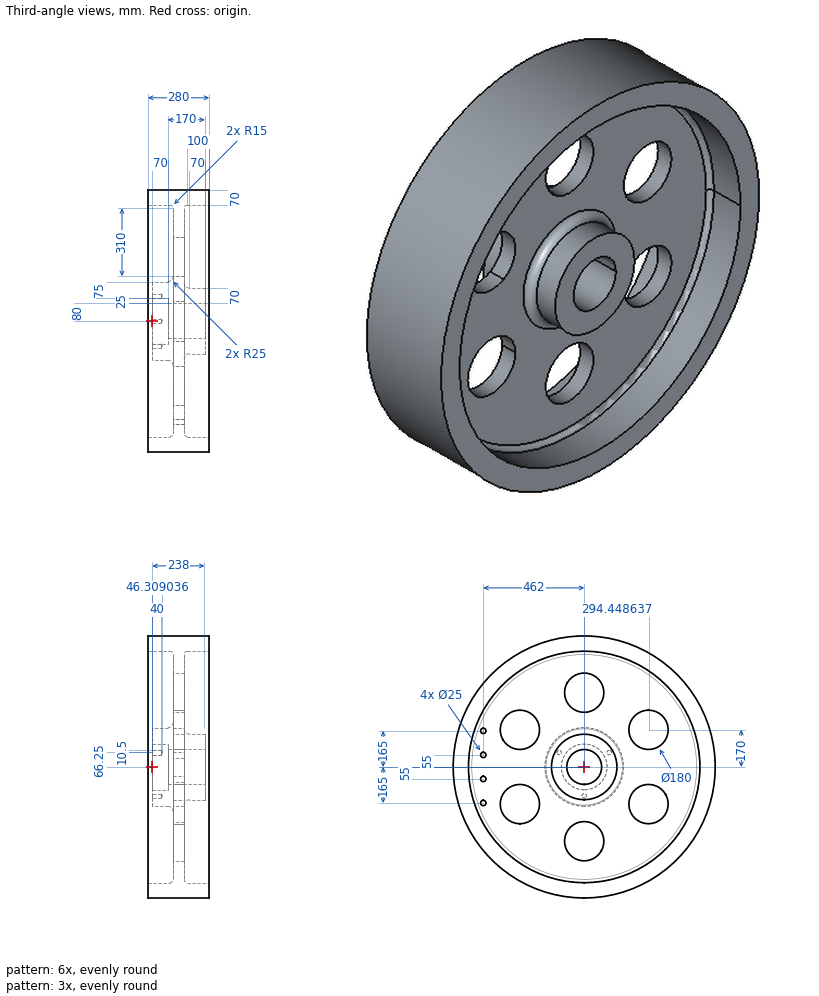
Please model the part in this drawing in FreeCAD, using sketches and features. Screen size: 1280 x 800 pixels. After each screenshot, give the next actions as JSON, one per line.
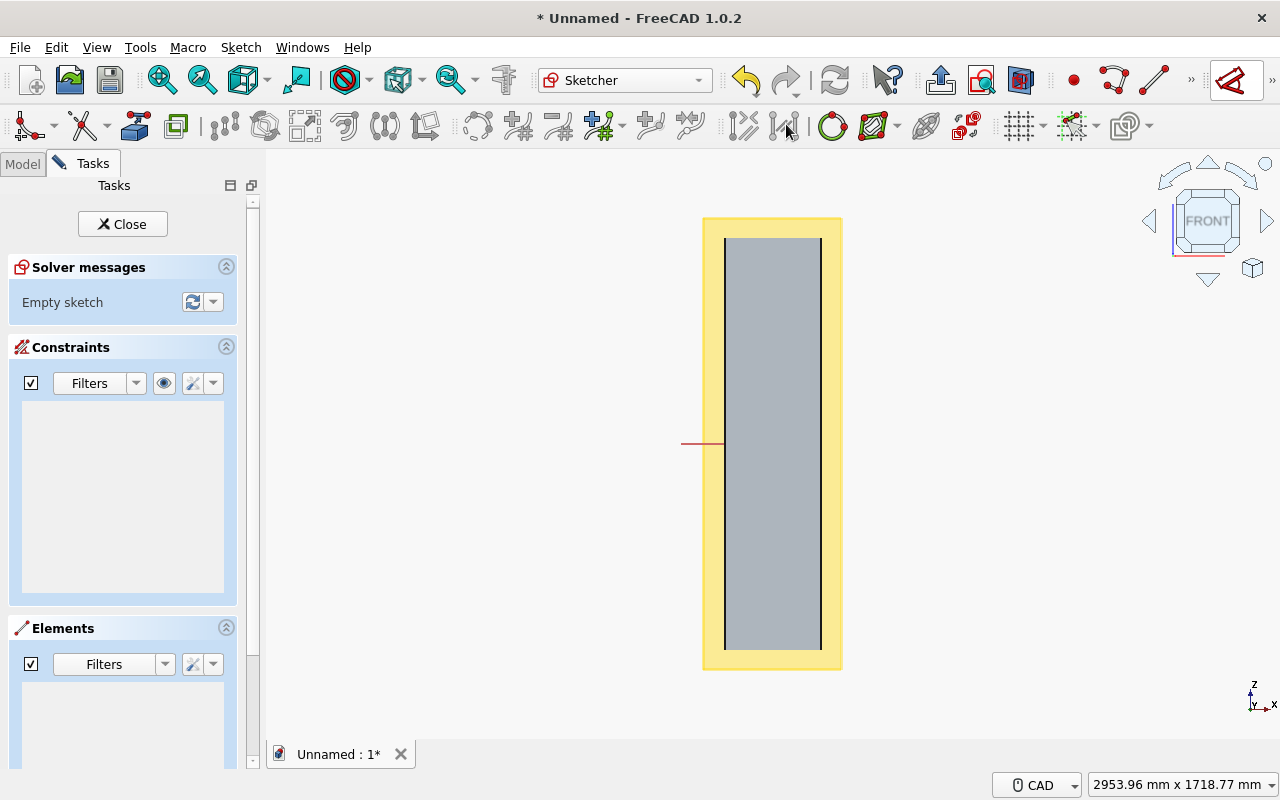
{"action": "left_click", "coordinate": [1022, 80]}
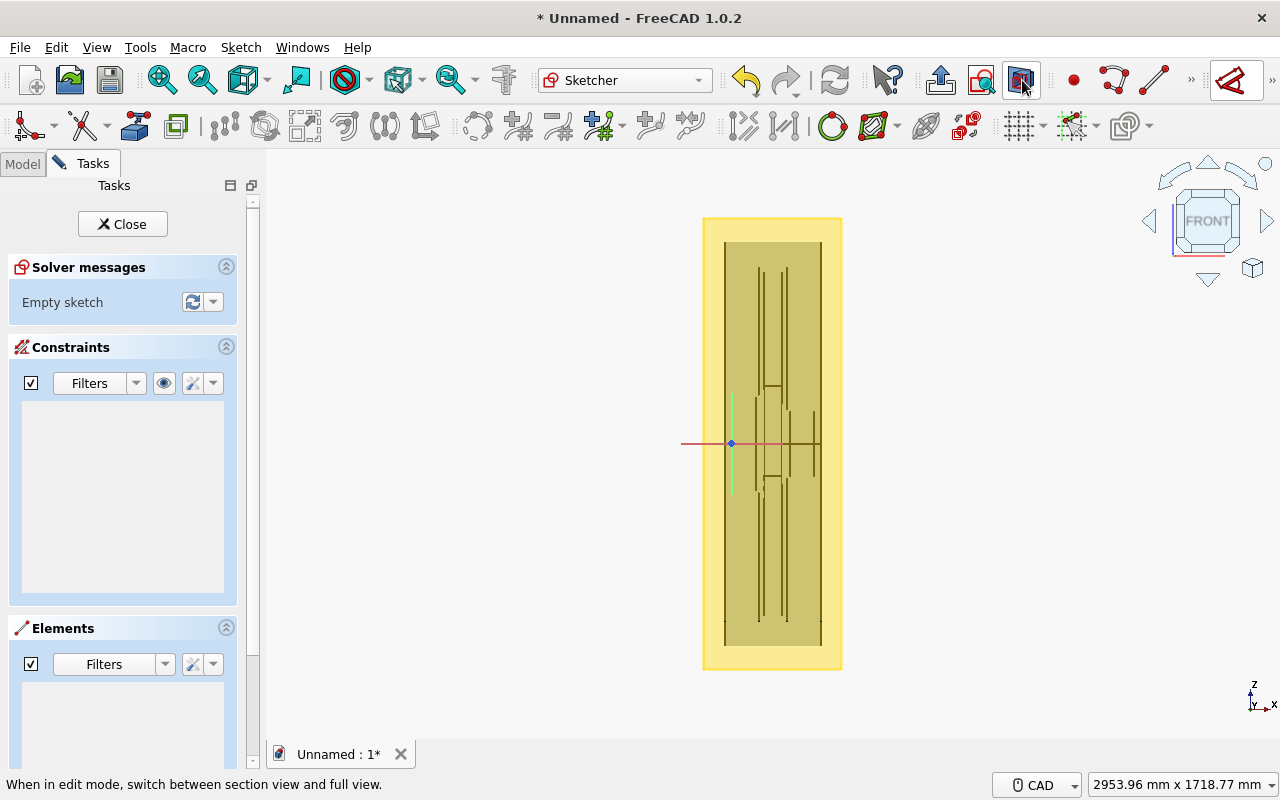
{"action": "scroll", "coordinate": [746, 430], "scroll_direction": "up", "scroll_amount": 13}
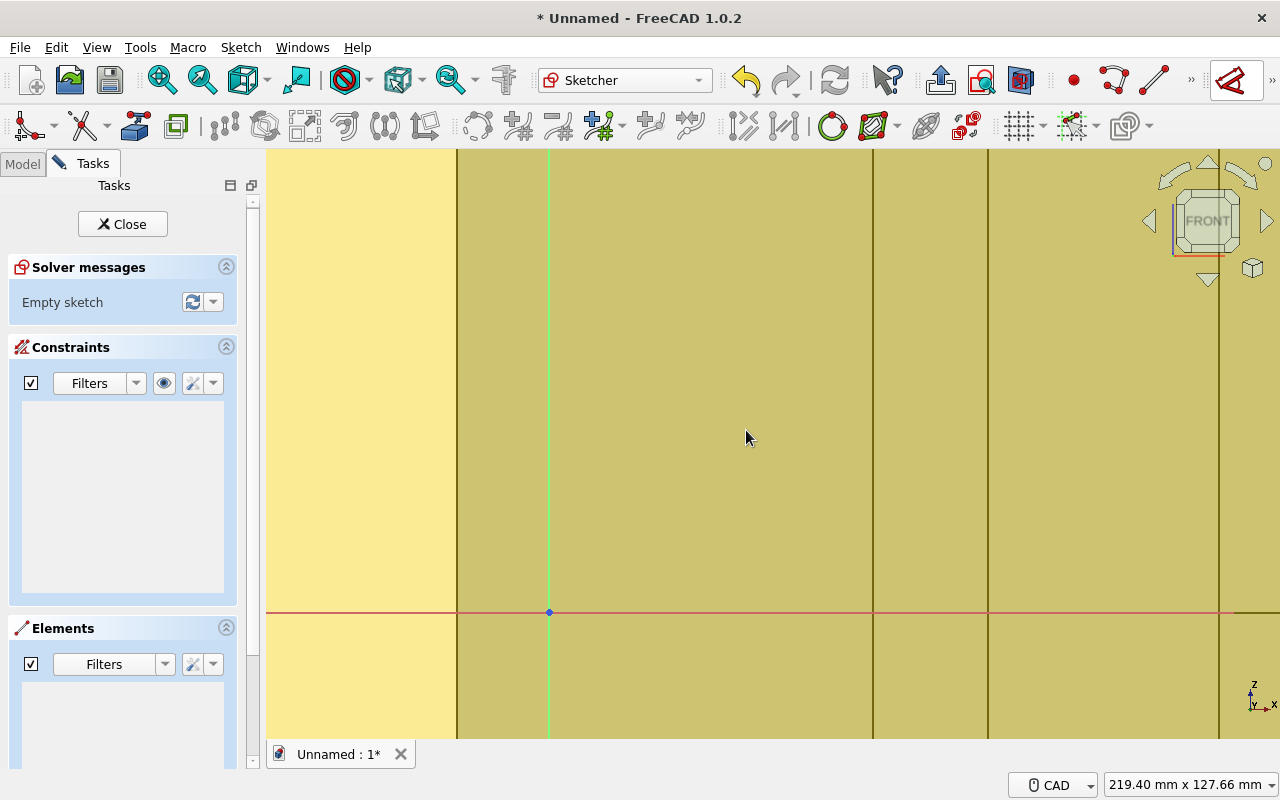
{"action": "left_click", "coordinate": [1114, 80]}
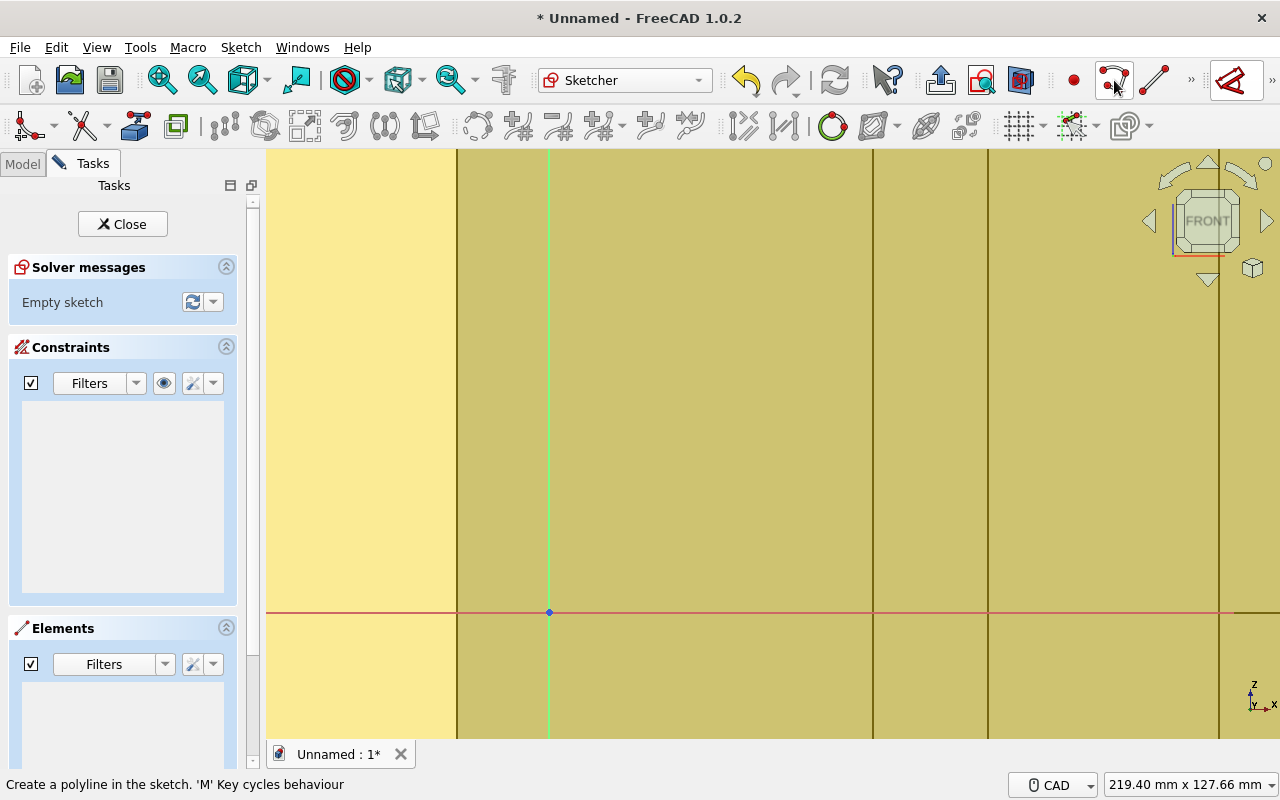
{"action": "left_click", "coordinate": [549, 306]}
{"action": "left_click", "coordinate": [558, 258]}
{"action": "left_click", "coordinate": [734, 258]}
{"action": "left_click", "coordinate": [763, 306]}
{"action": "left_click", "coordinate": [549, 307]}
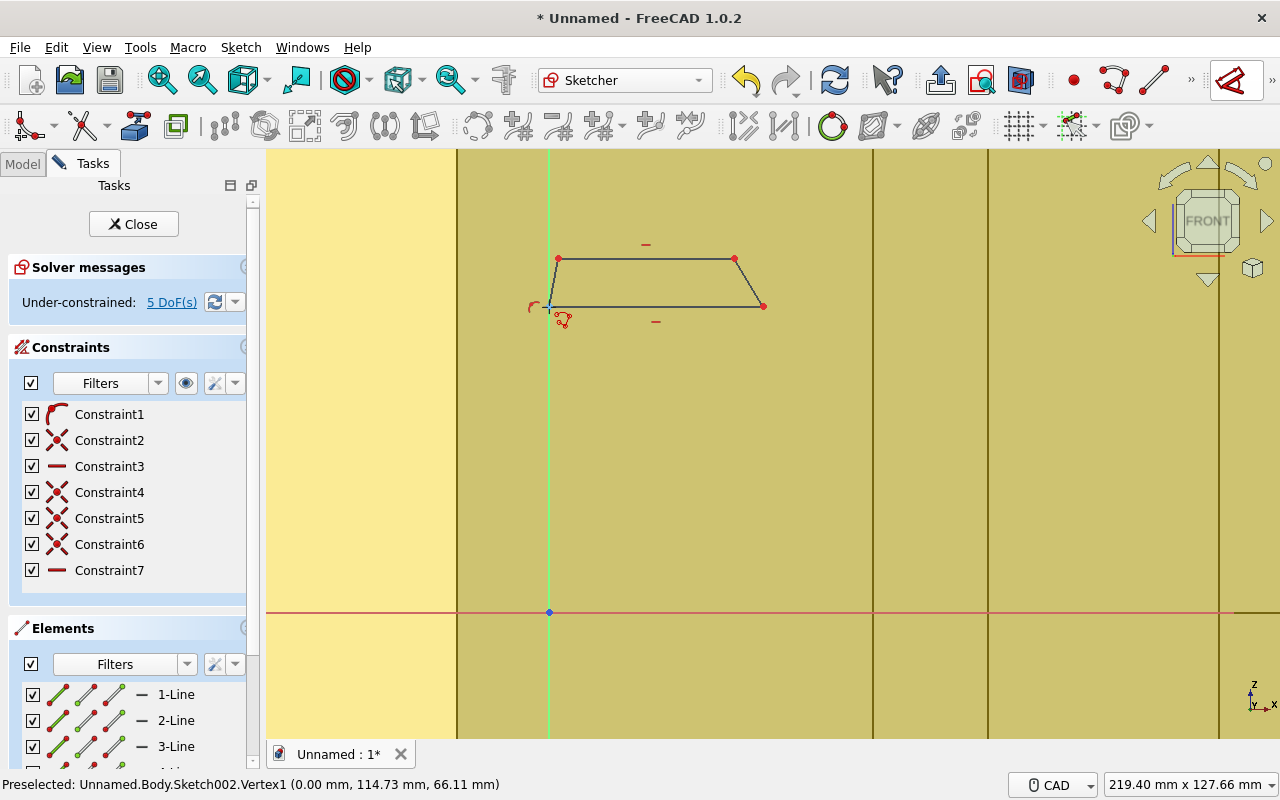
{"action": "left_click", "coordinate": [1154, 80]}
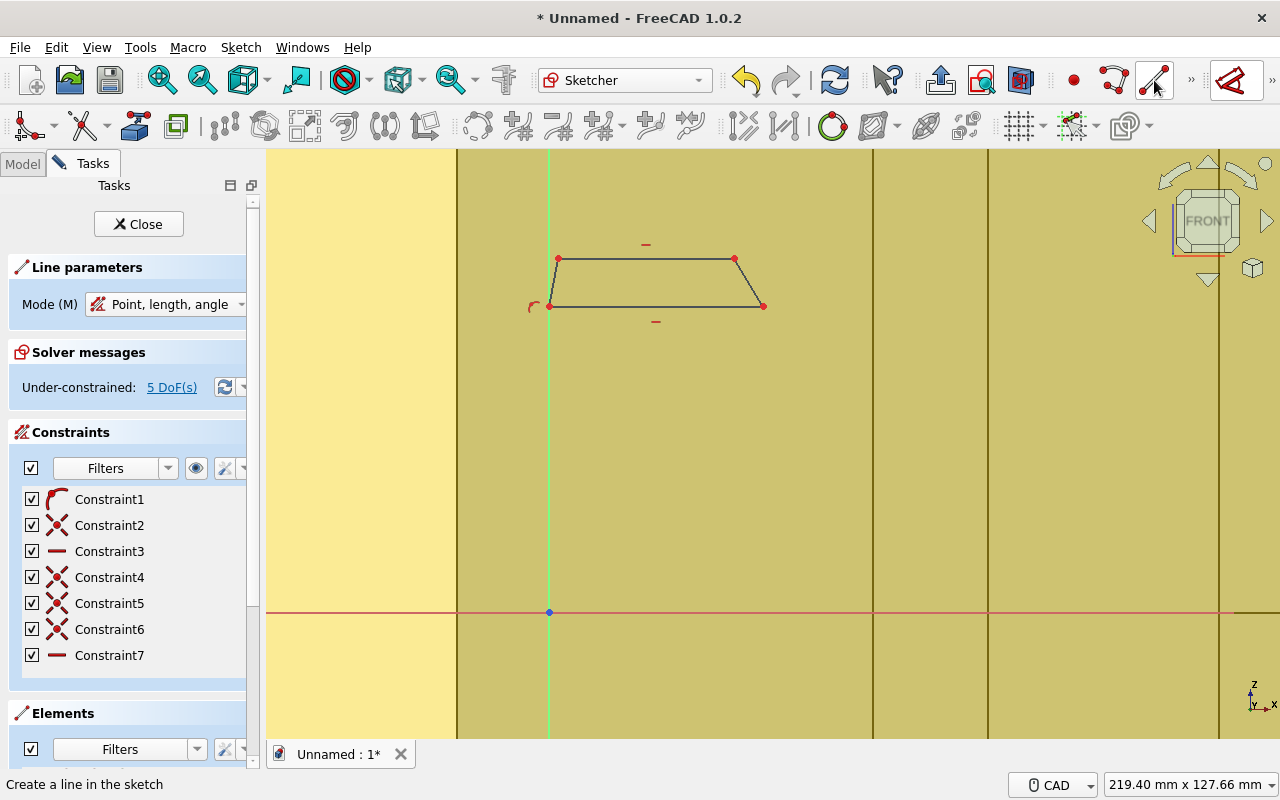
{"action": "left_click", "coordinate": [784, 306]}
{"action": "left_click", "coordinate": [849, 306]}
{"action": "key", "text": "Escape"}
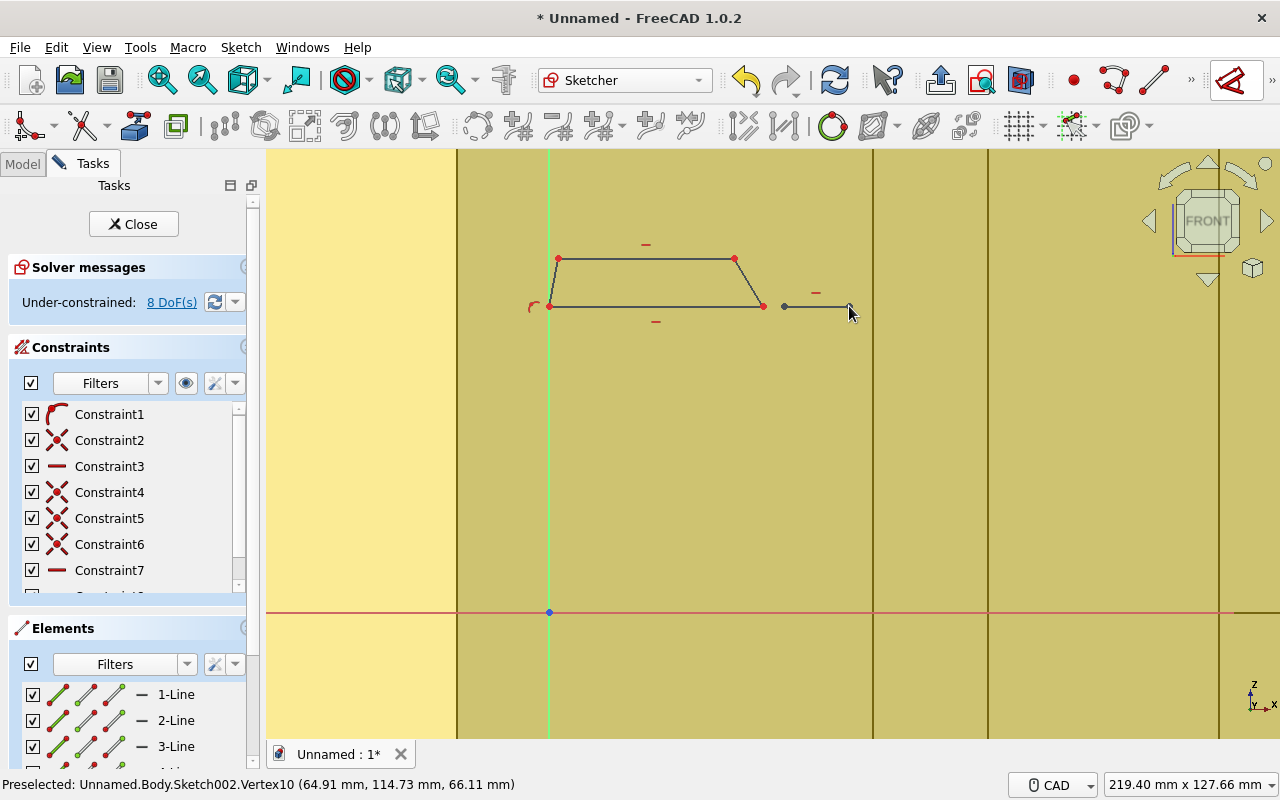
{"action": "left_click", "coordinate": [803, 307]}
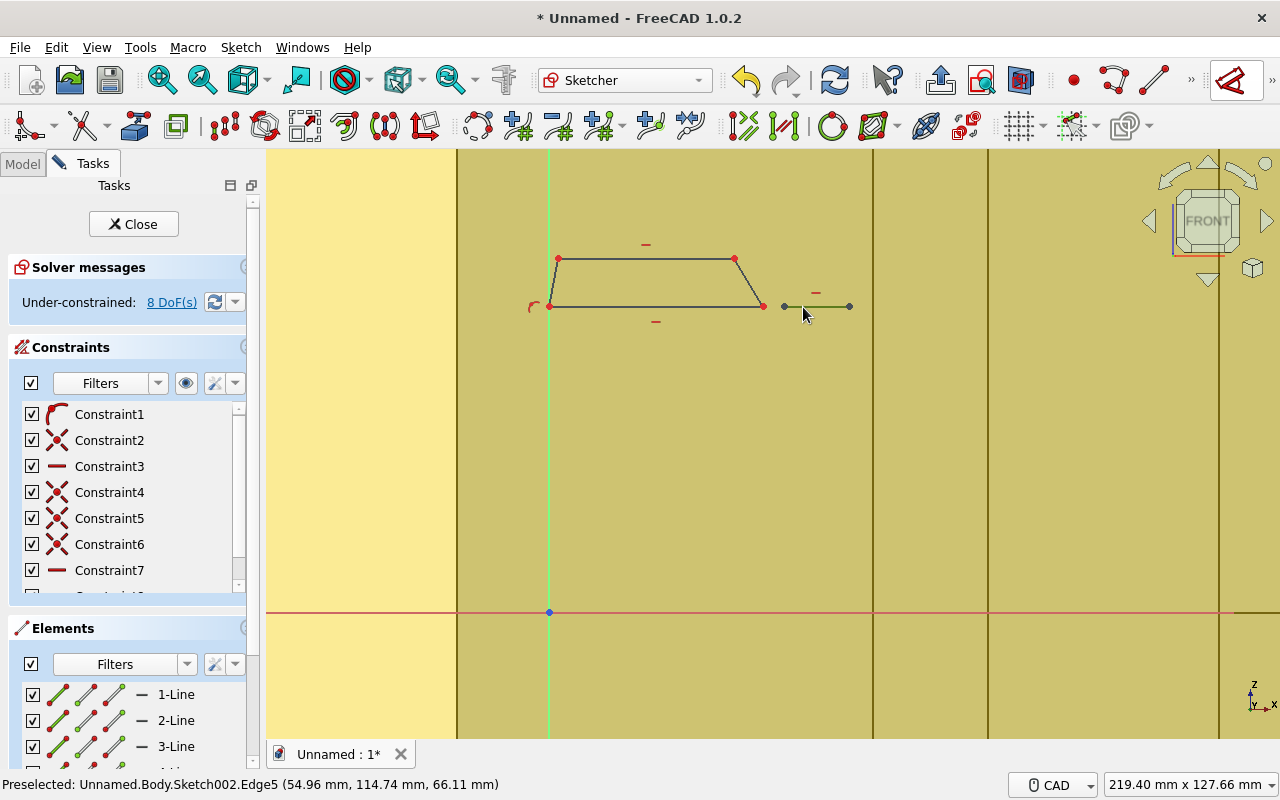
{"action": "key", "text": "g n"}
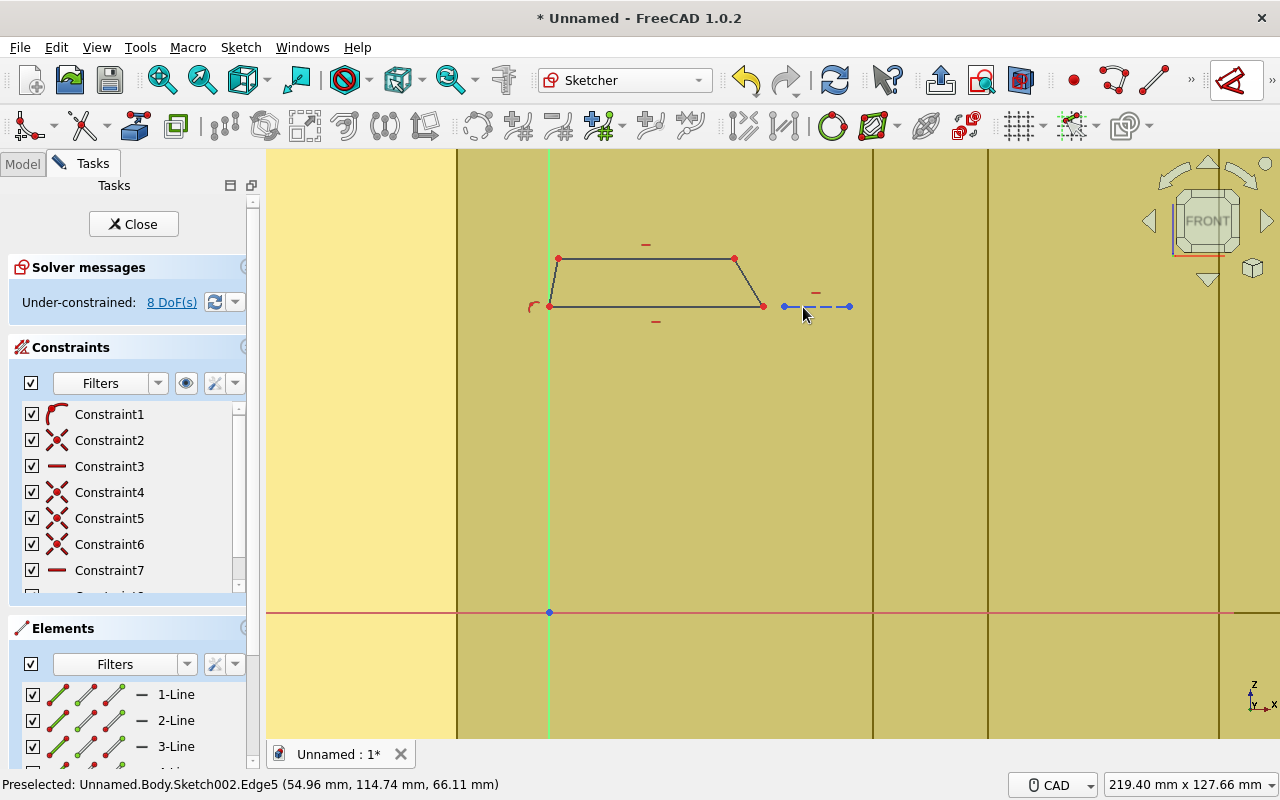
{"action": "left_click", "coordinate": [552, 293]}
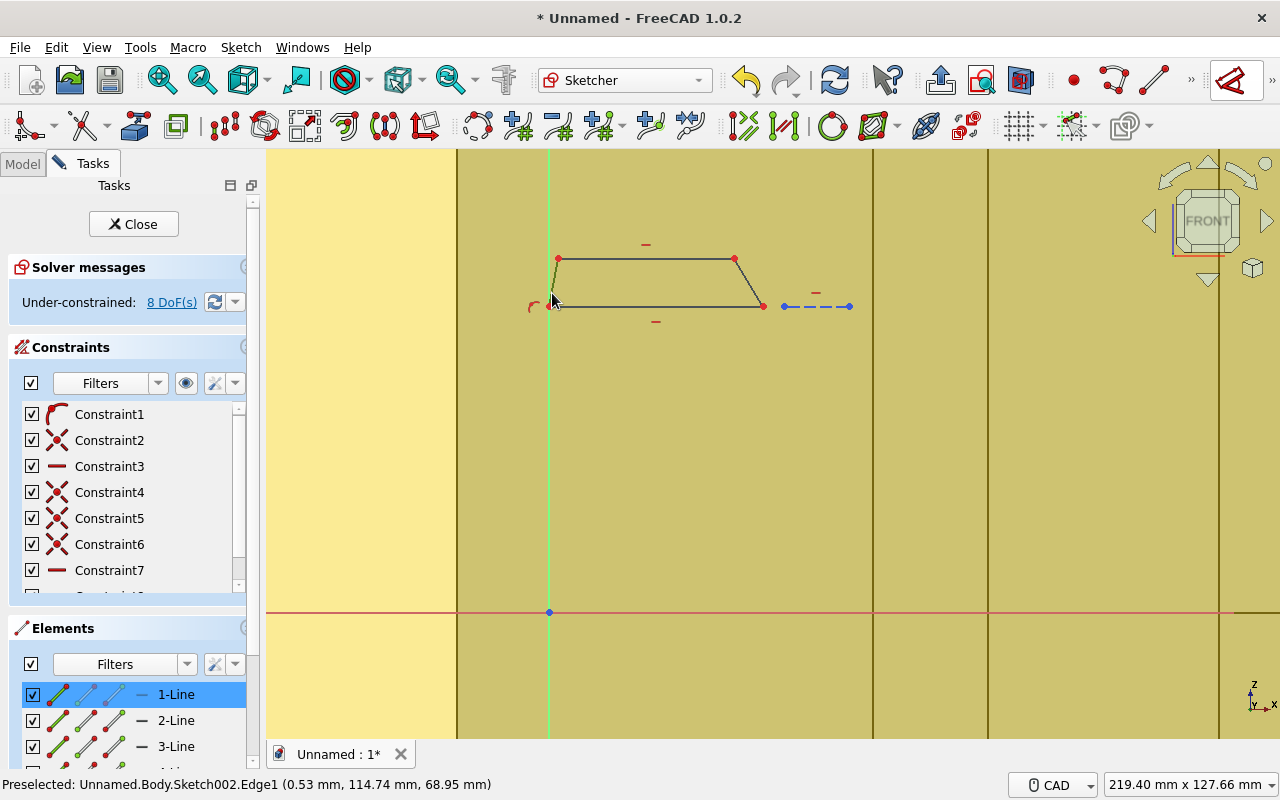
{"action": "key", "text": "v"}